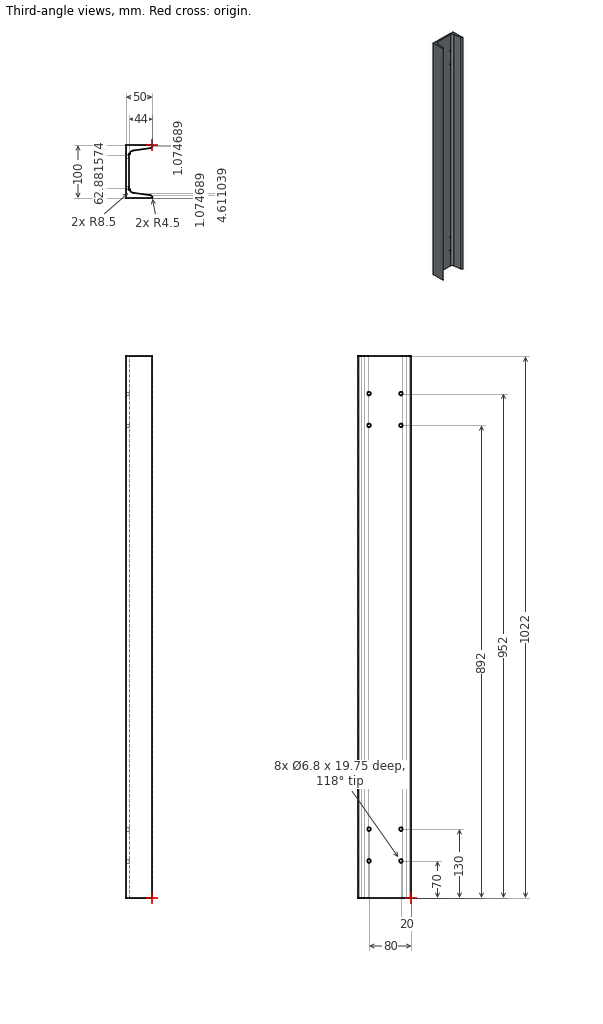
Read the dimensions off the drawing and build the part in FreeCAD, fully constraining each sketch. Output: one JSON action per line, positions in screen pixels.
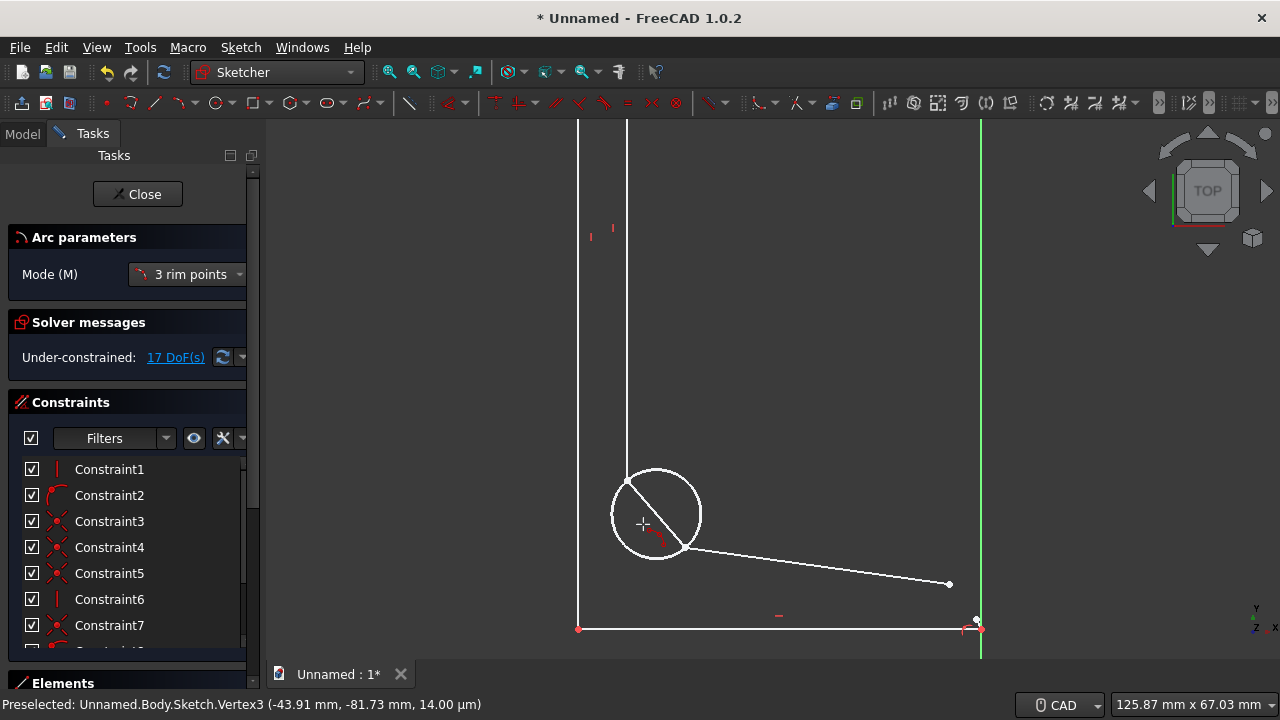
{"action": "left_click", "coordinate": [643, 523]}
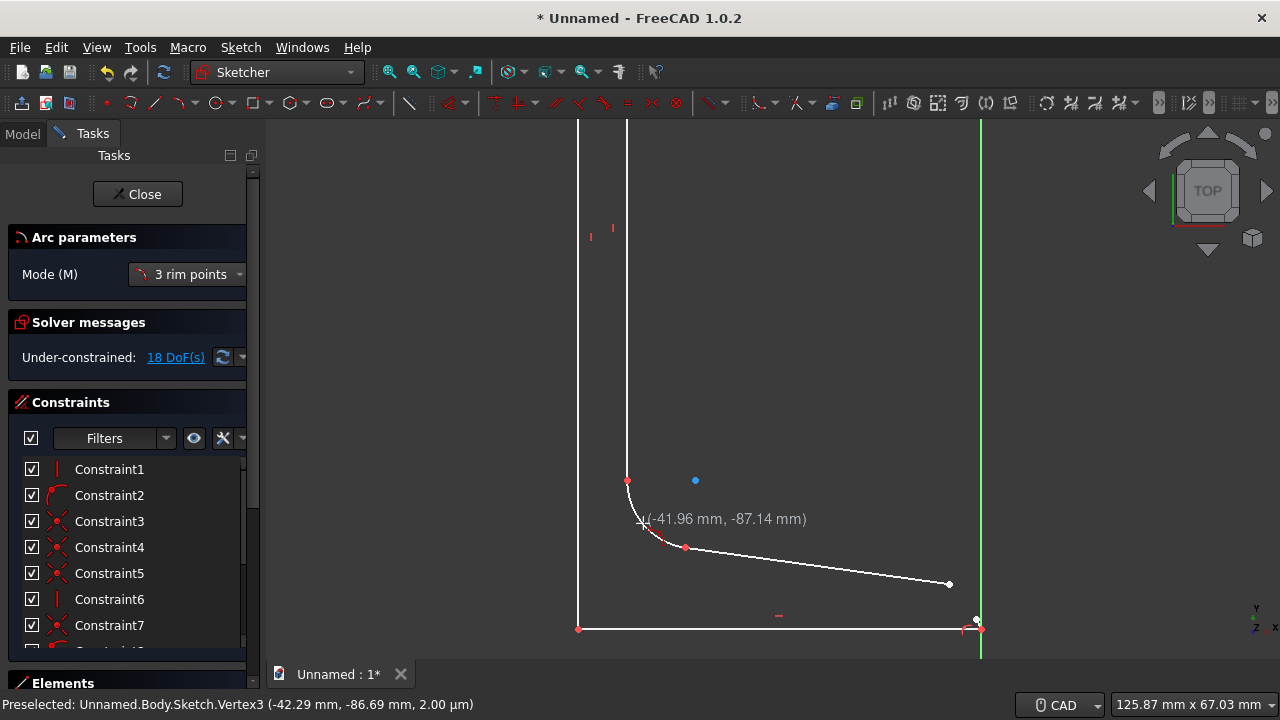
{"action": "scroll", "coordinate": [643, 523], "scroll_direction": "down", "scroll_amount": 4}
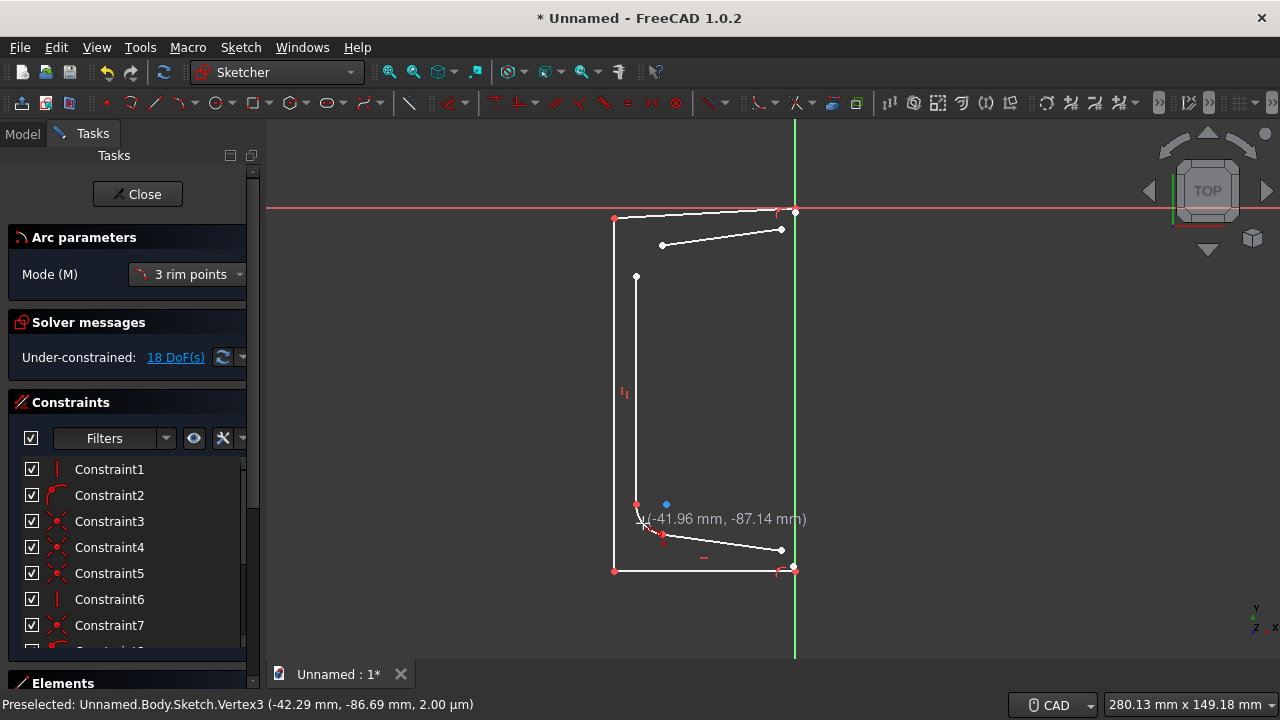
{"action": "left_click", "coordinate": [636, 277]}
{"action": "left_click", "coordinate": [662, 246]}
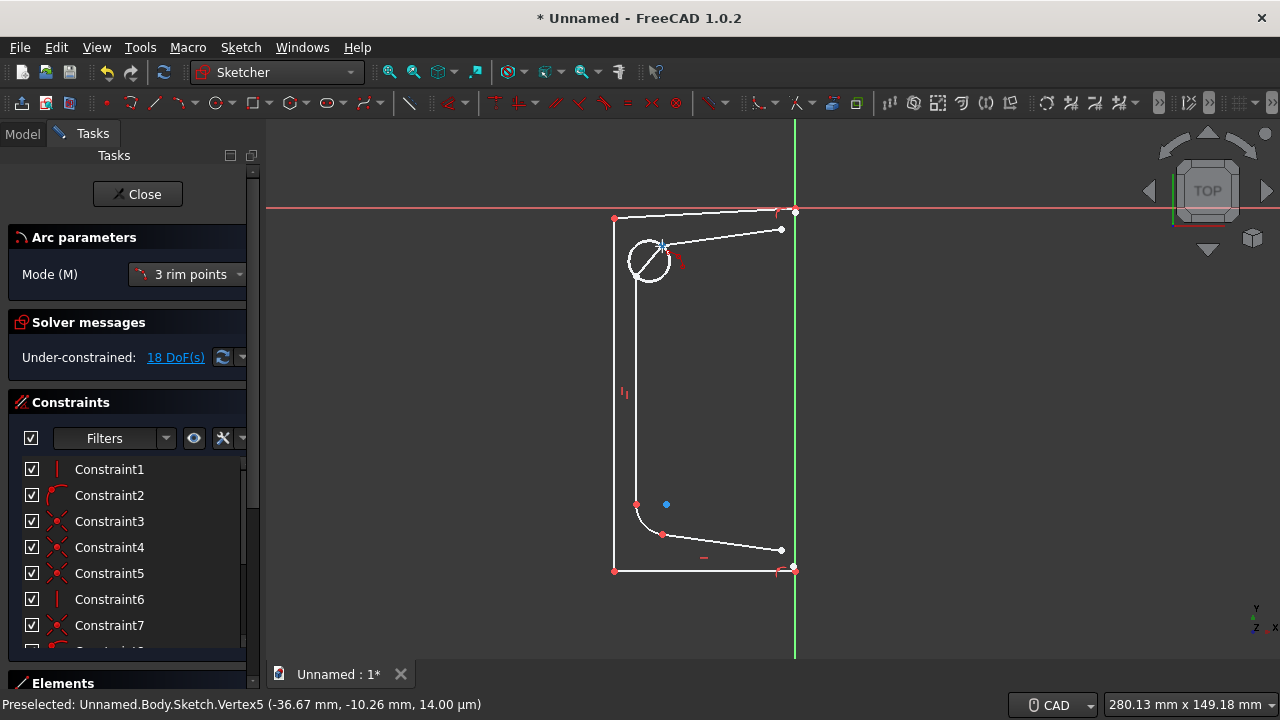
{"action": "scroll", "coordinate": [643, 255], "scroll_direction": "up", "scroll_amount": 4}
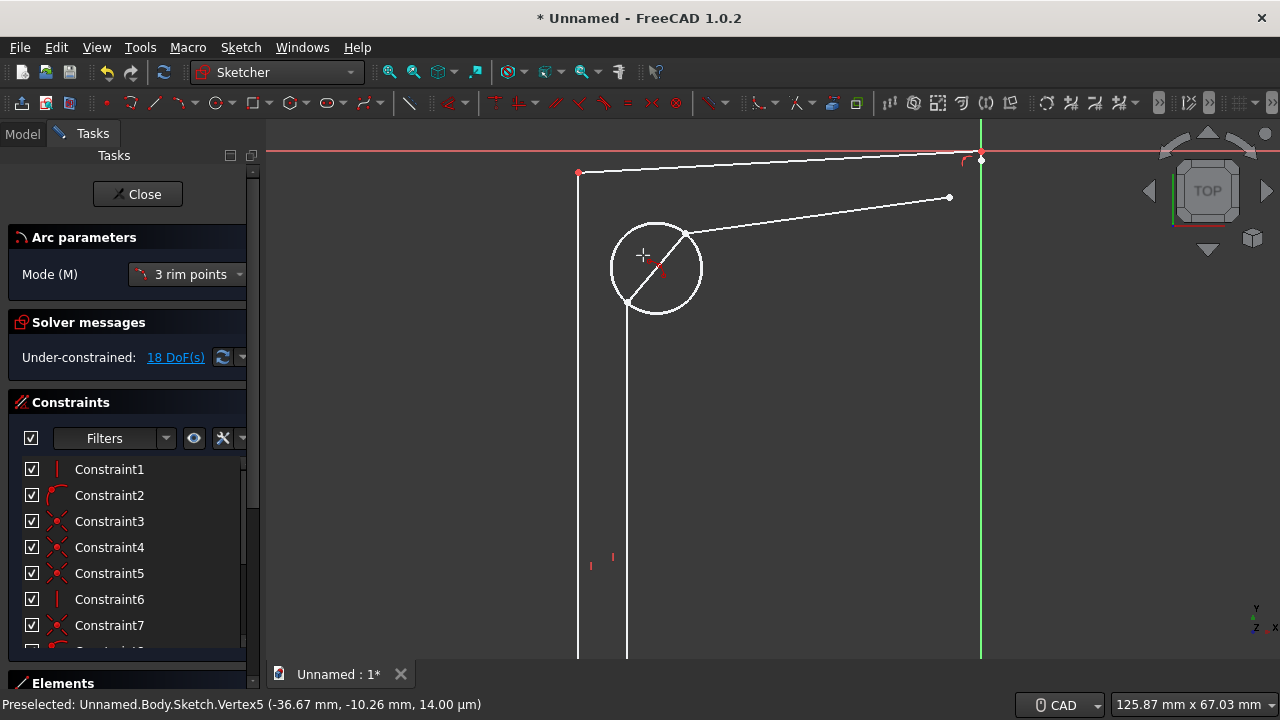
{"action": "left_click", "coordinate": [643, 256]}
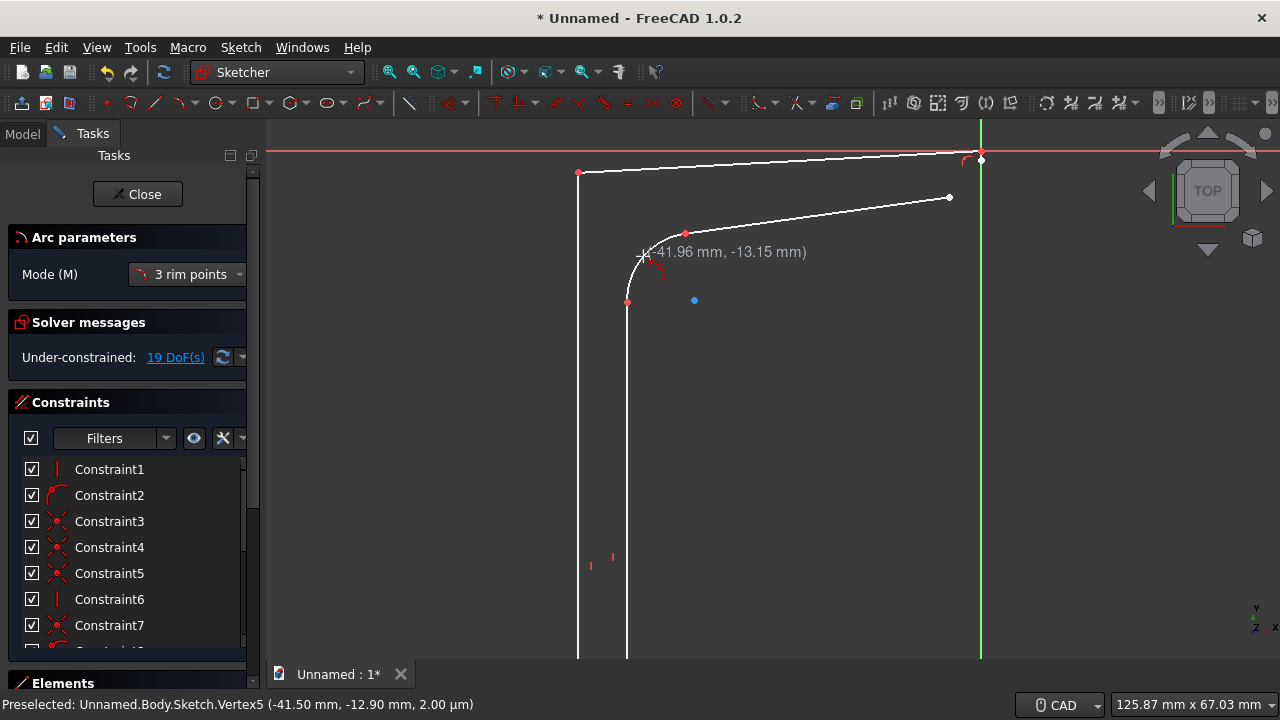
{"action": "left_click", "coordinate": [950, 197]}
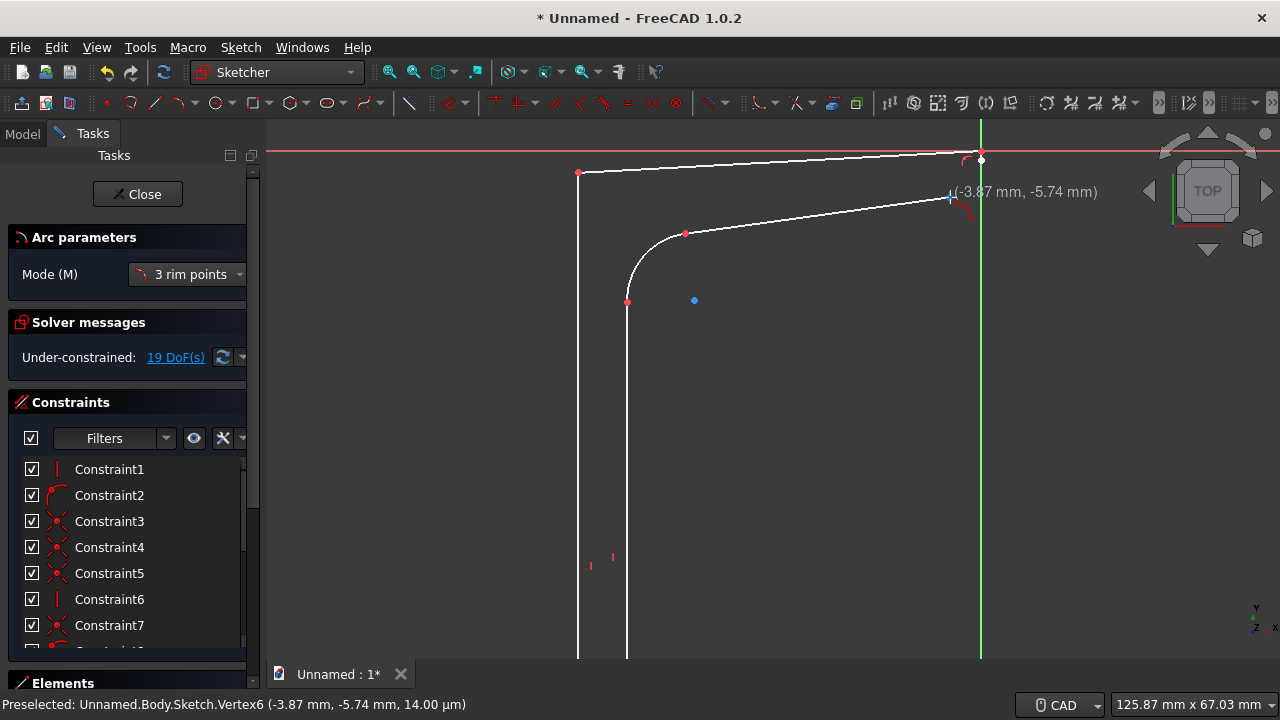
{"action": "scroll", "coordinate": [981, 160], "scroll_direction": "up", "scroll_amount": 7}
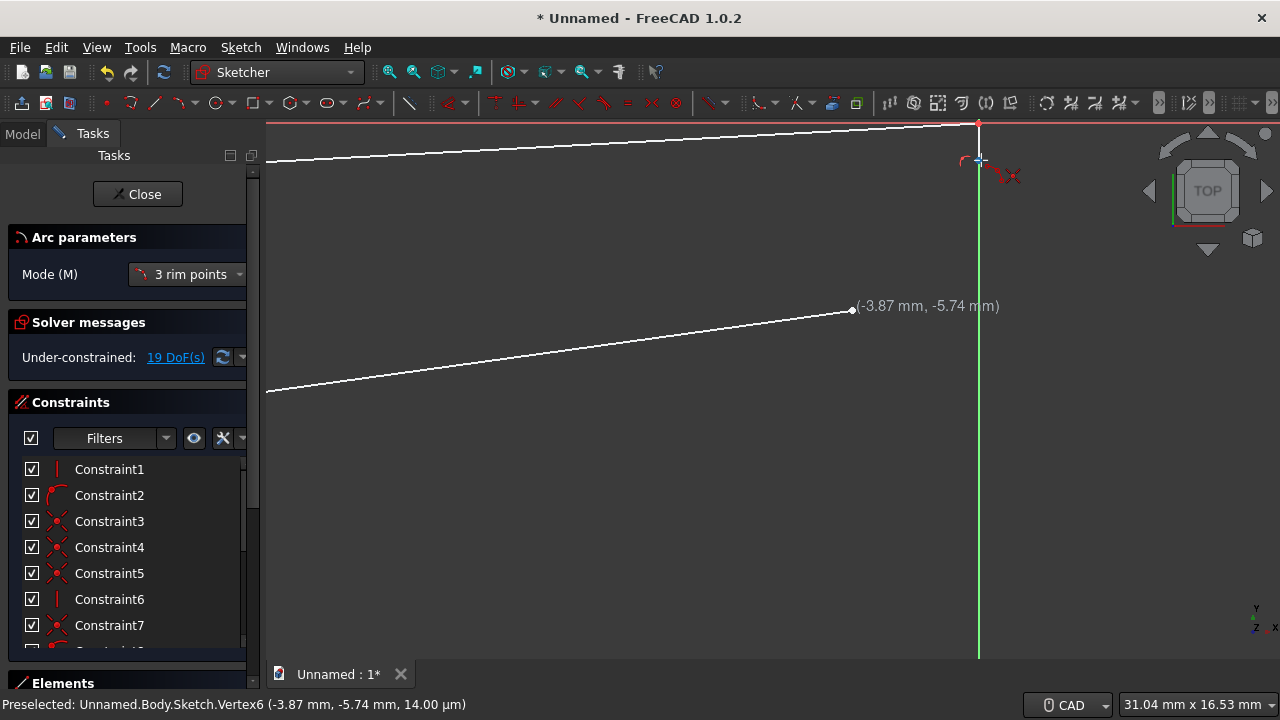
{"action": "left_click", "coordinate": [979, 161]}
{"action": "left_click", "coordinate": [943, 255]}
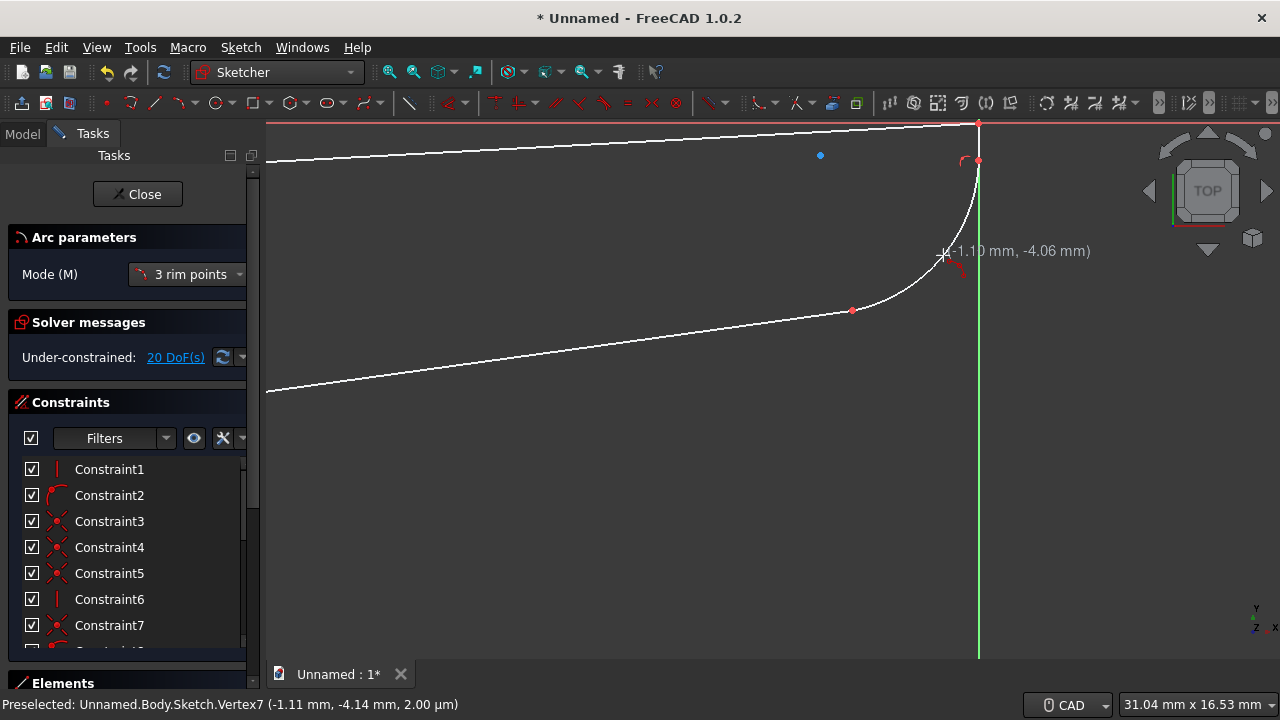
{"action": "scroll", "coordinate": [772, 219], "scroll_direction": "down", "scroll_amount": 11}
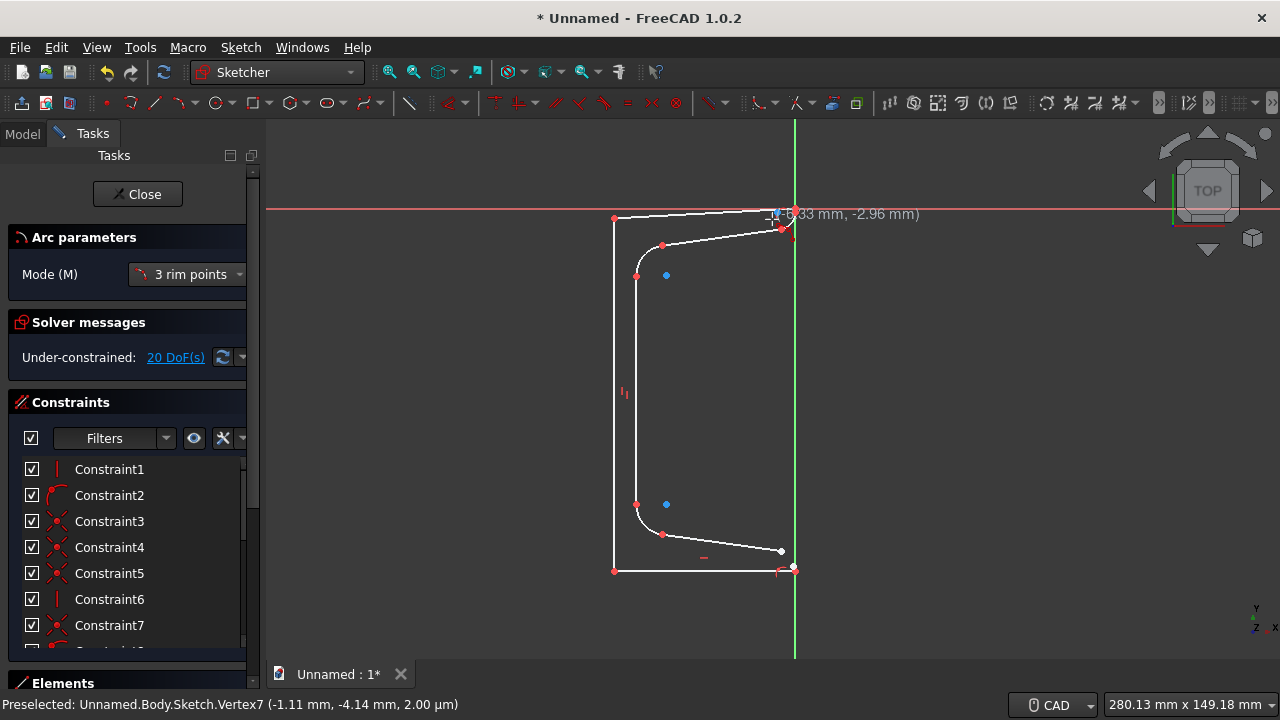
{"action": "scroll", "coordinate": [795, 567], "scroll_direction": "up", "scroll_amount": 11}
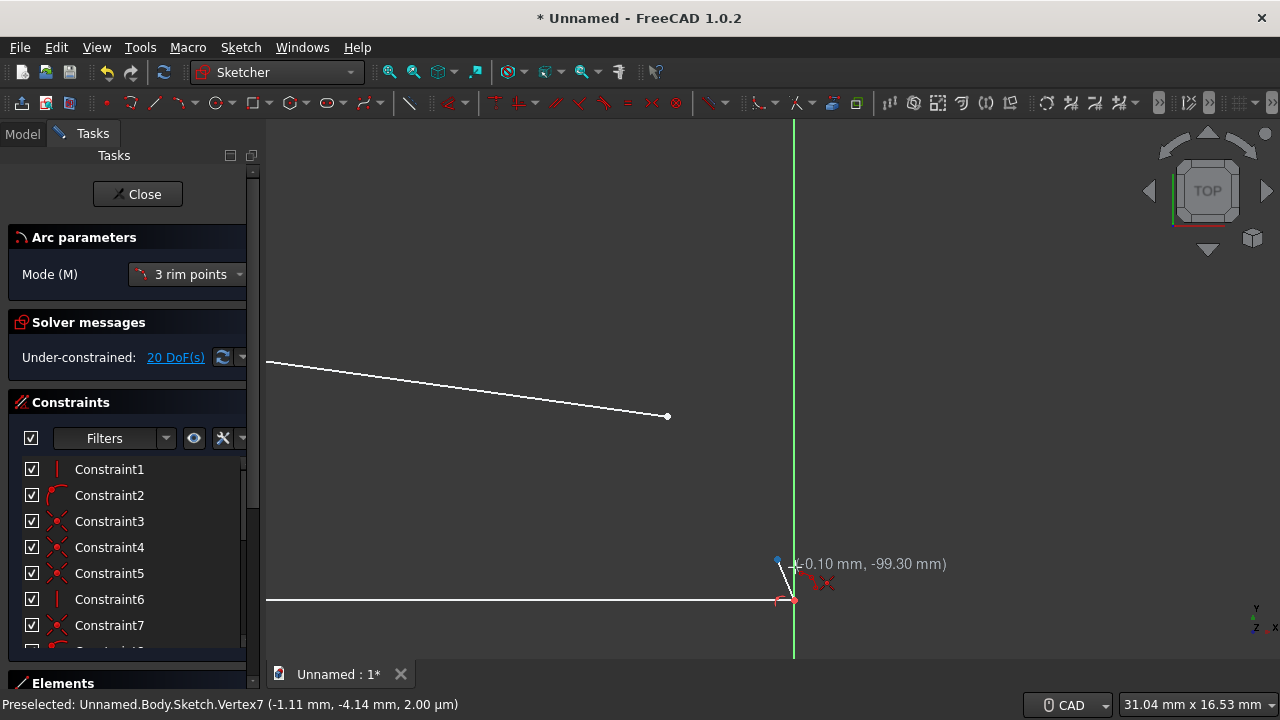
{"action": "left_click", "coordinate": [777, 559]}